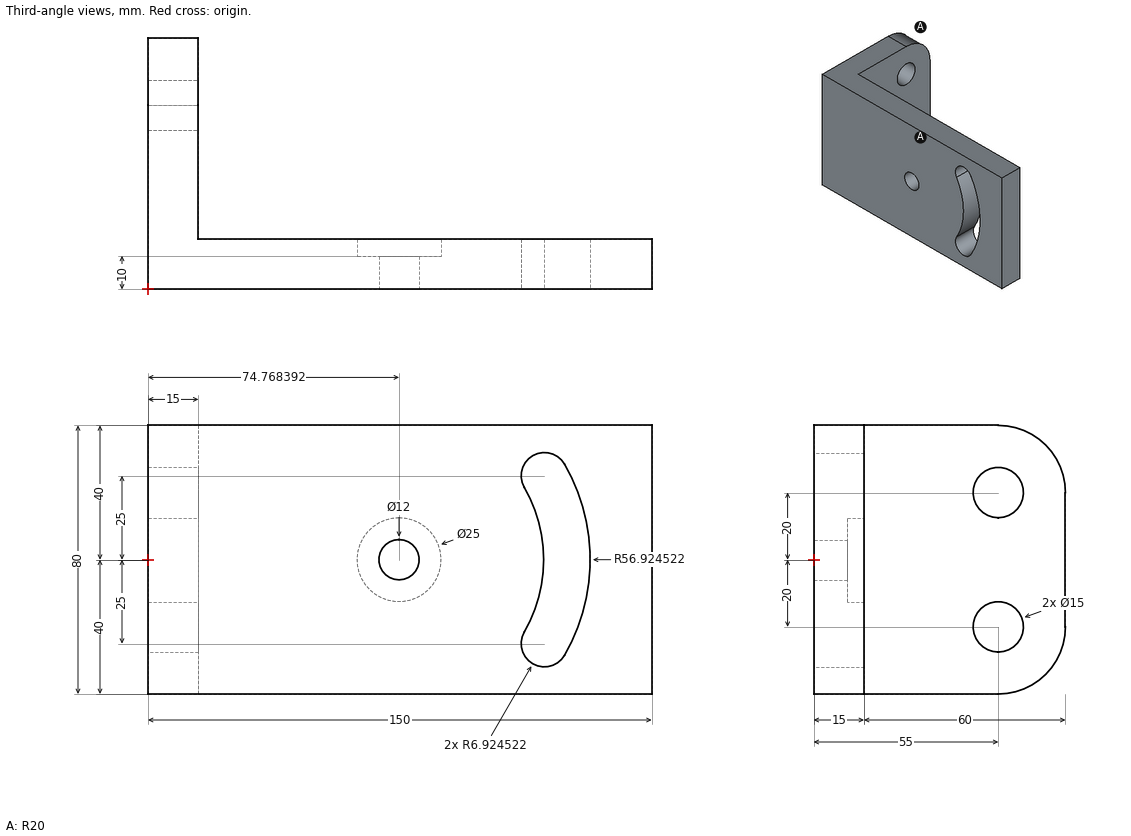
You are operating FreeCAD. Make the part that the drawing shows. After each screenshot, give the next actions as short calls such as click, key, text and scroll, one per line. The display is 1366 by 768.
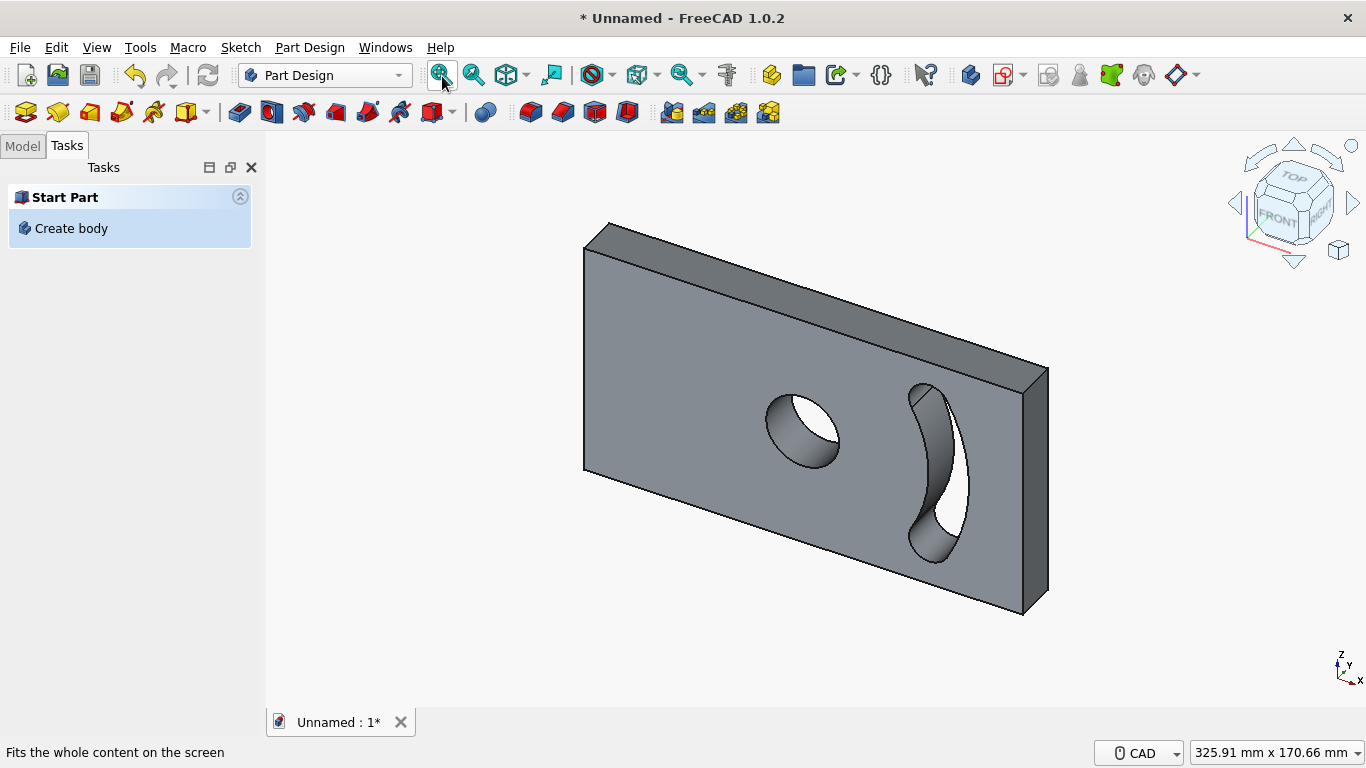
click(1004, 76)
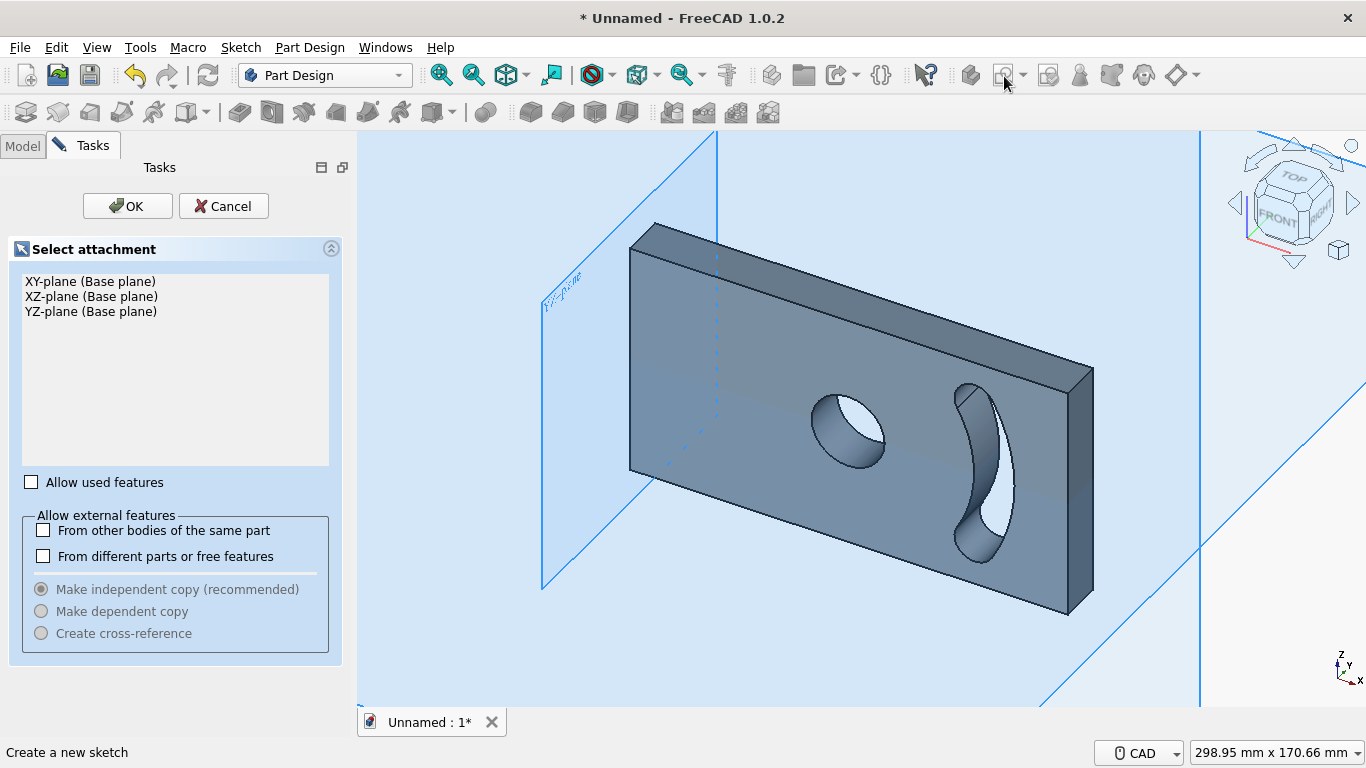
click(82, 296)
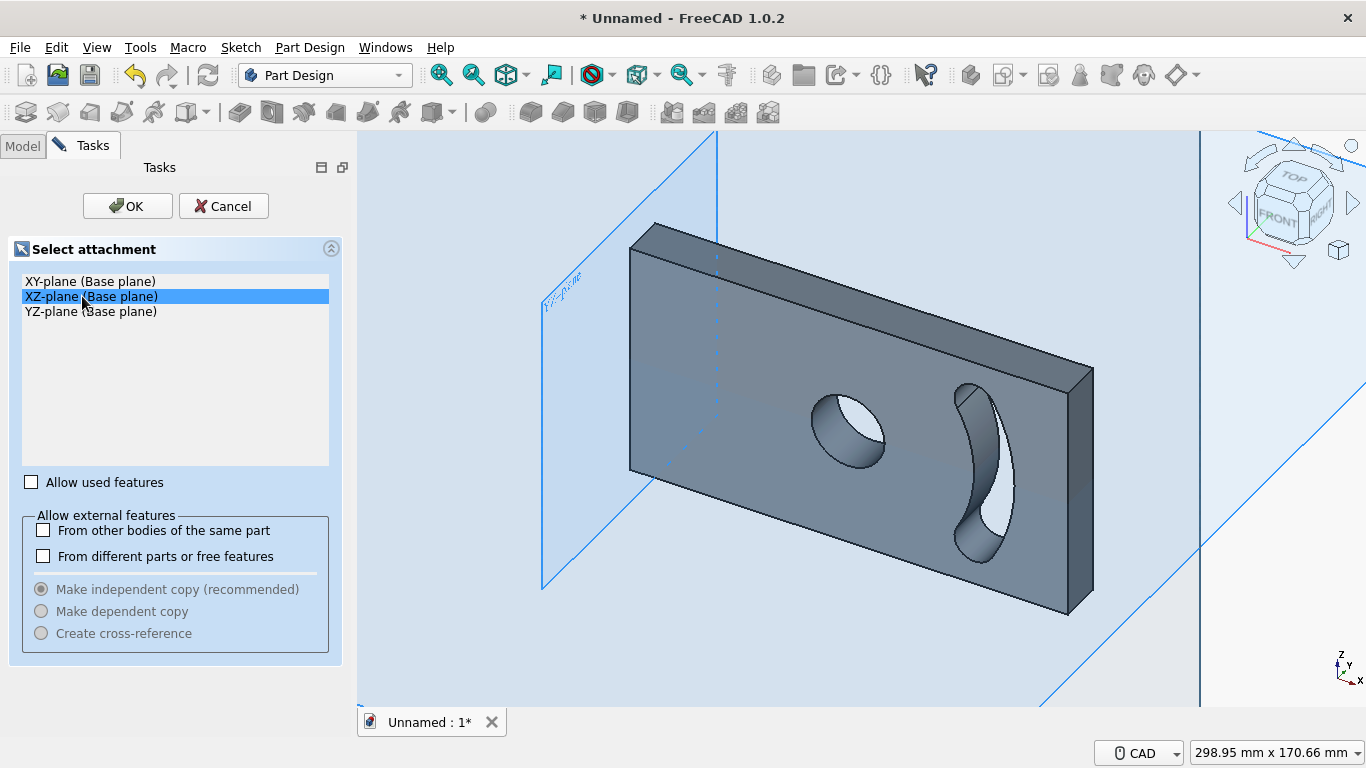
click(128, 206)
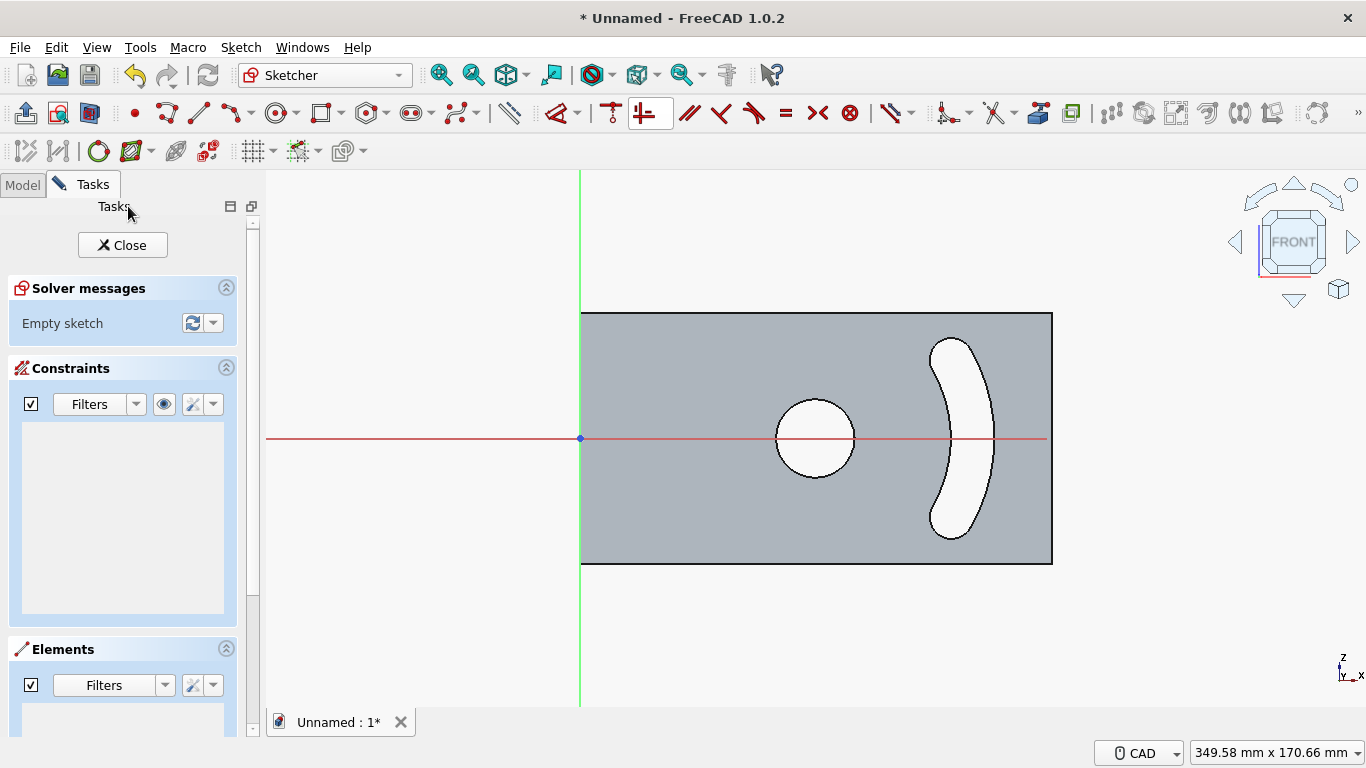
scroll(837, 439, up, 7)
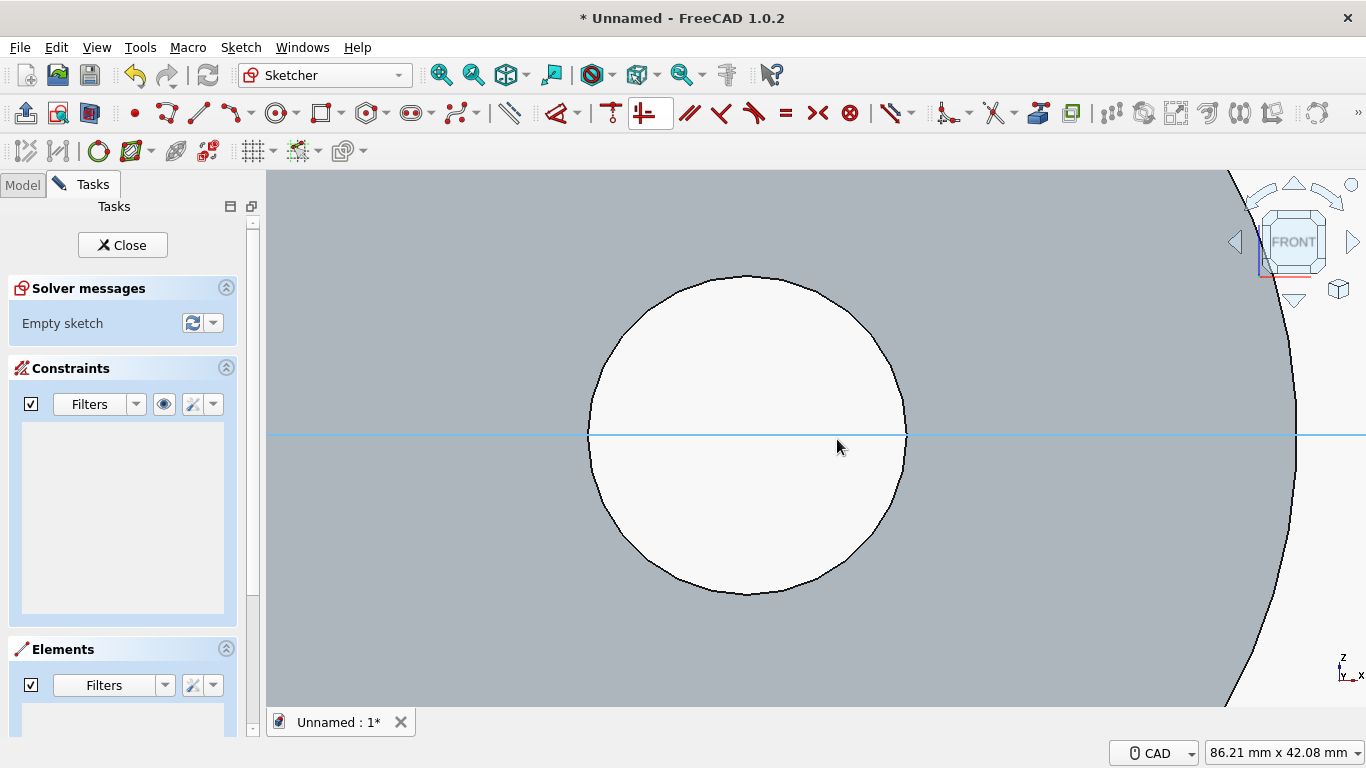
key(g)
key(c)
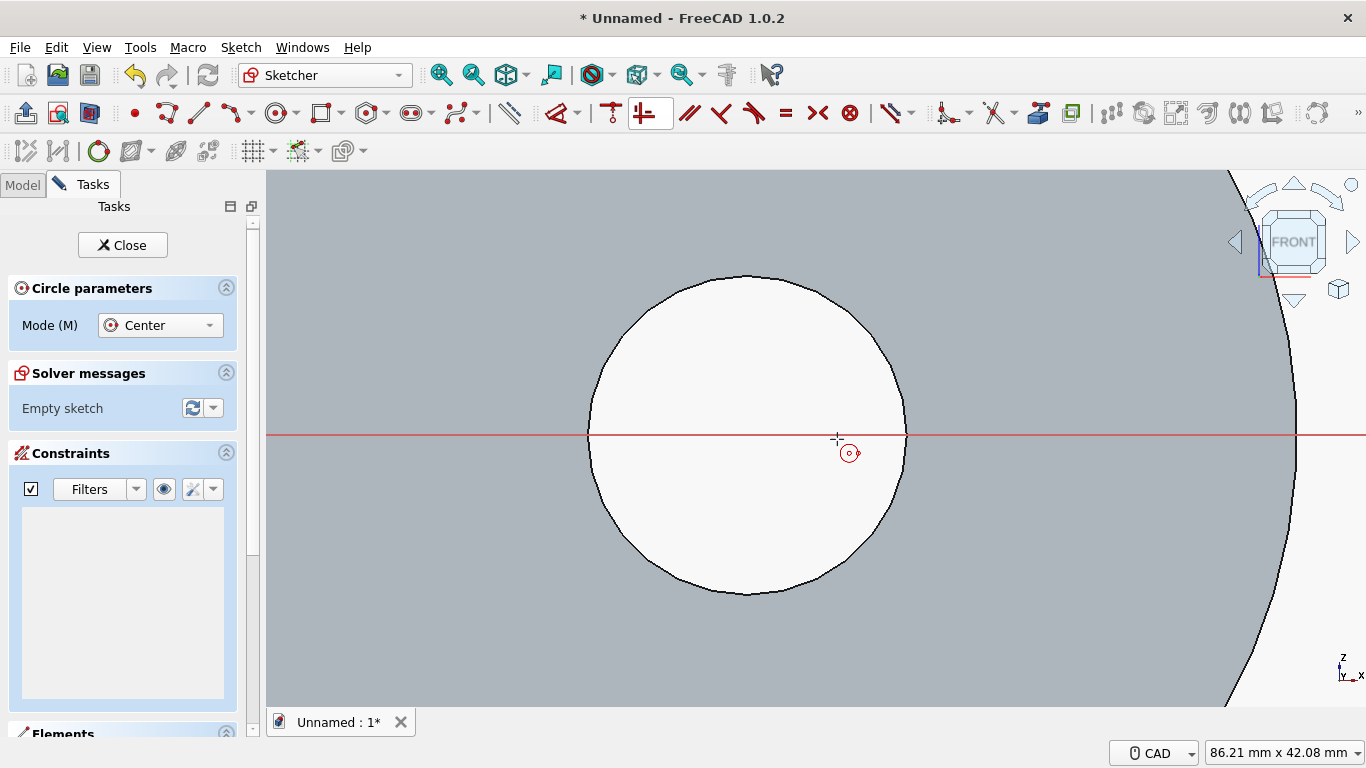
click(747, 435)
click(860, 323)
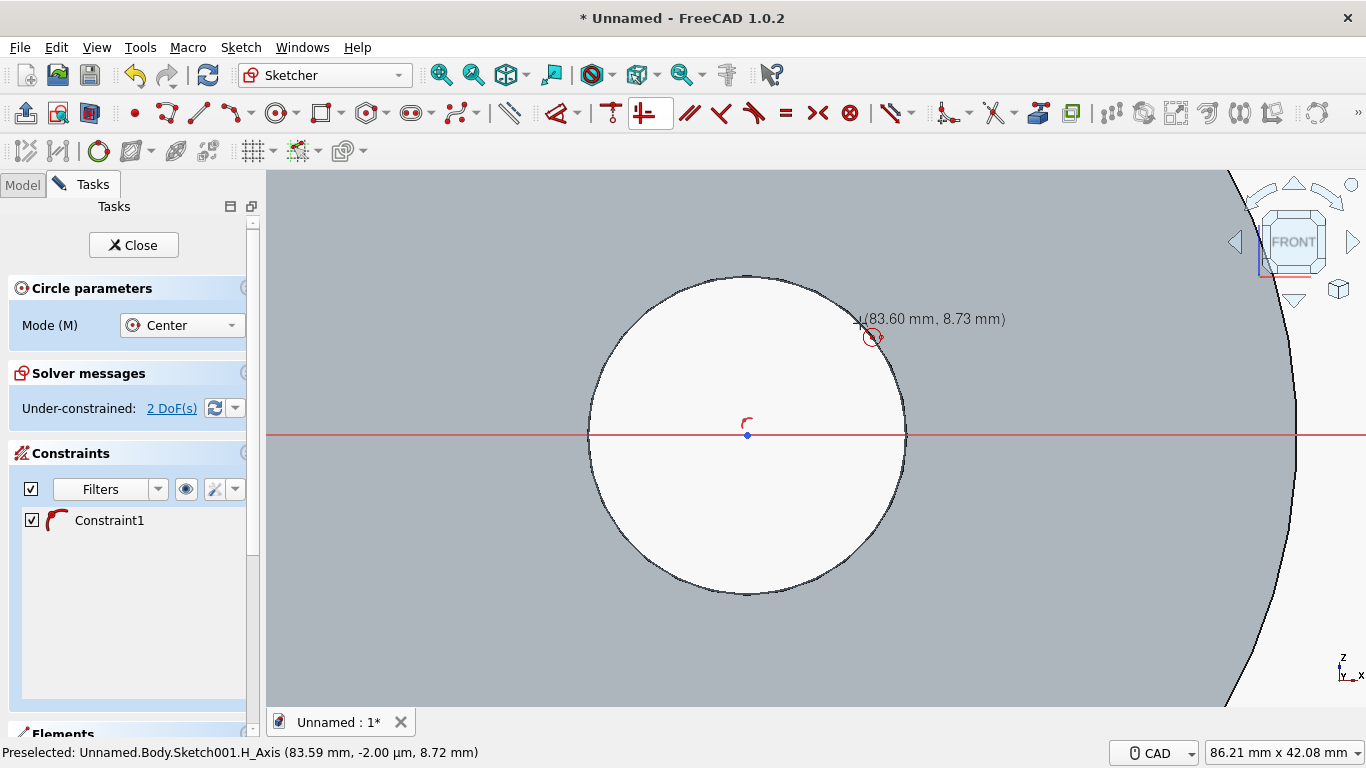
click(747, 435)
click(801, 381)
key(Escape)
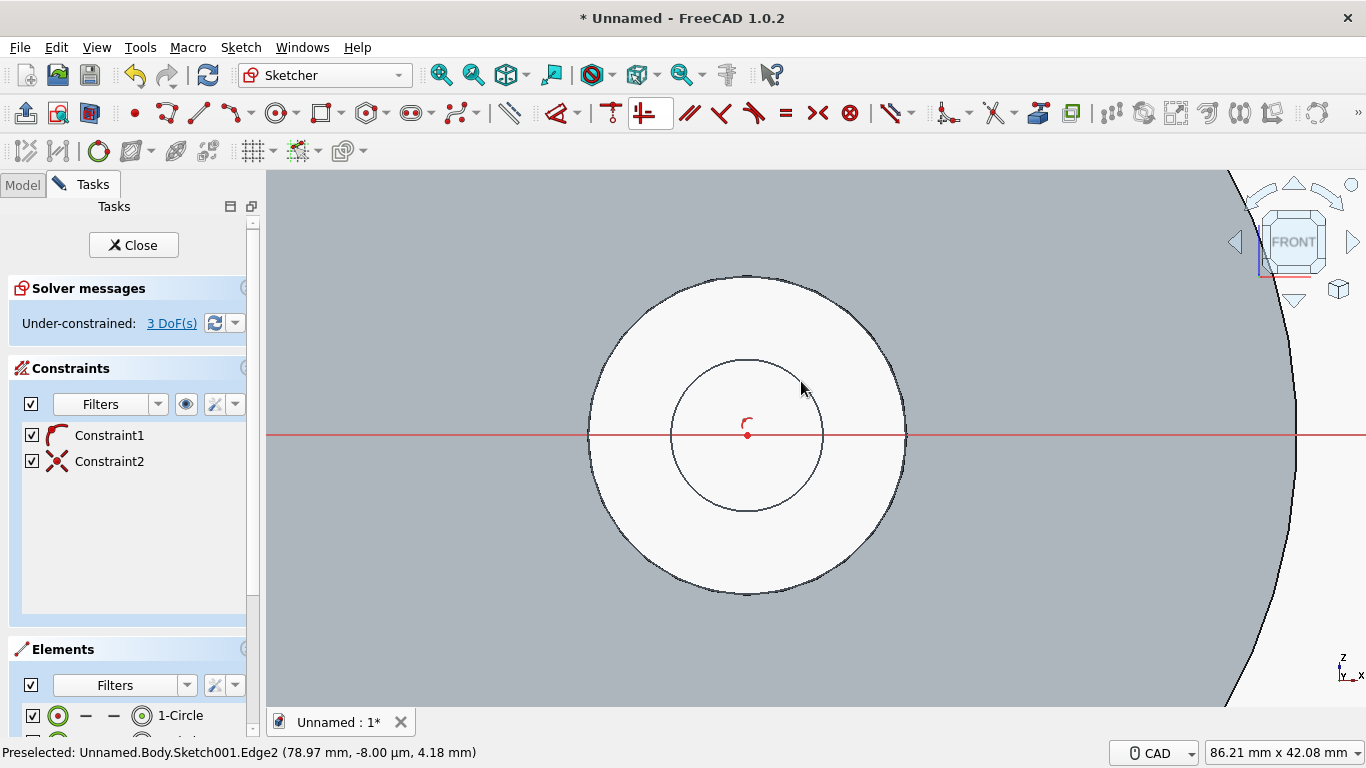
click(556, 114)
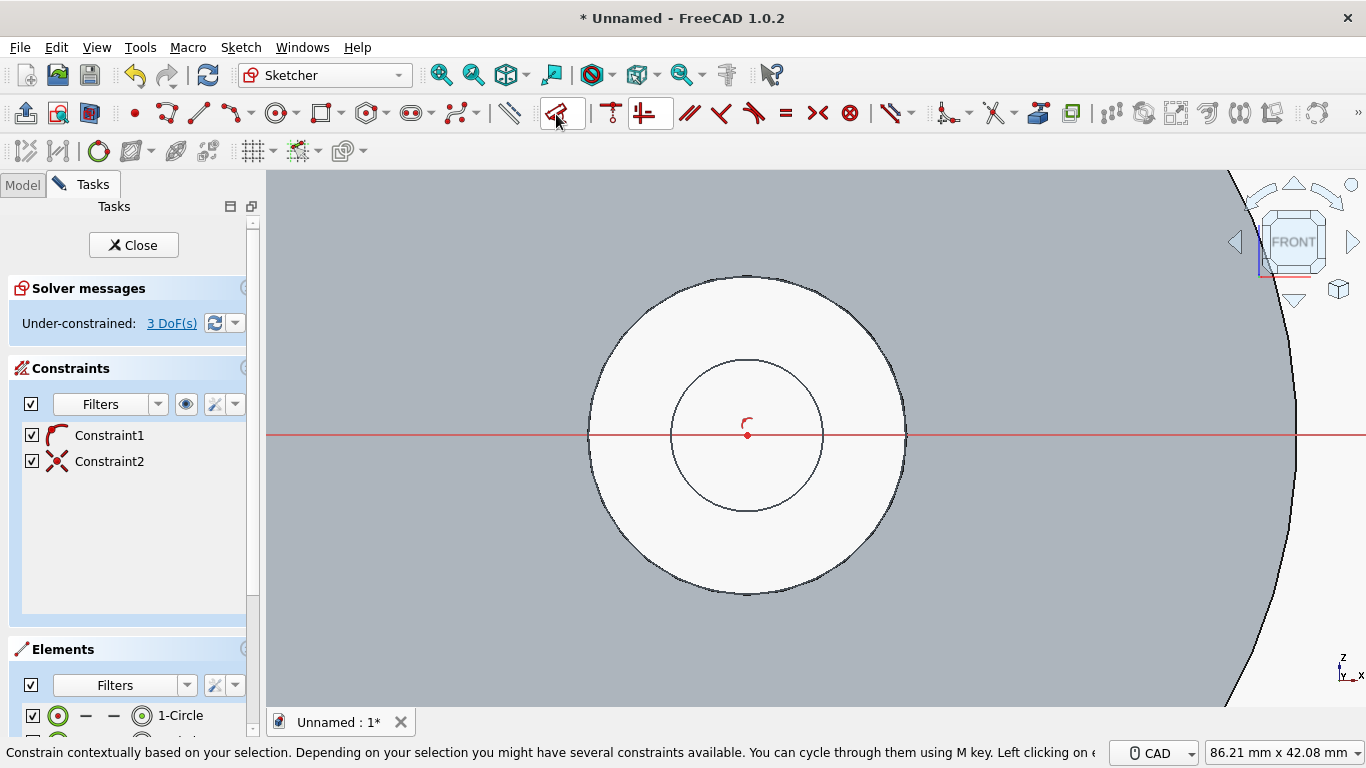
click(859, 323)
click(882, 300)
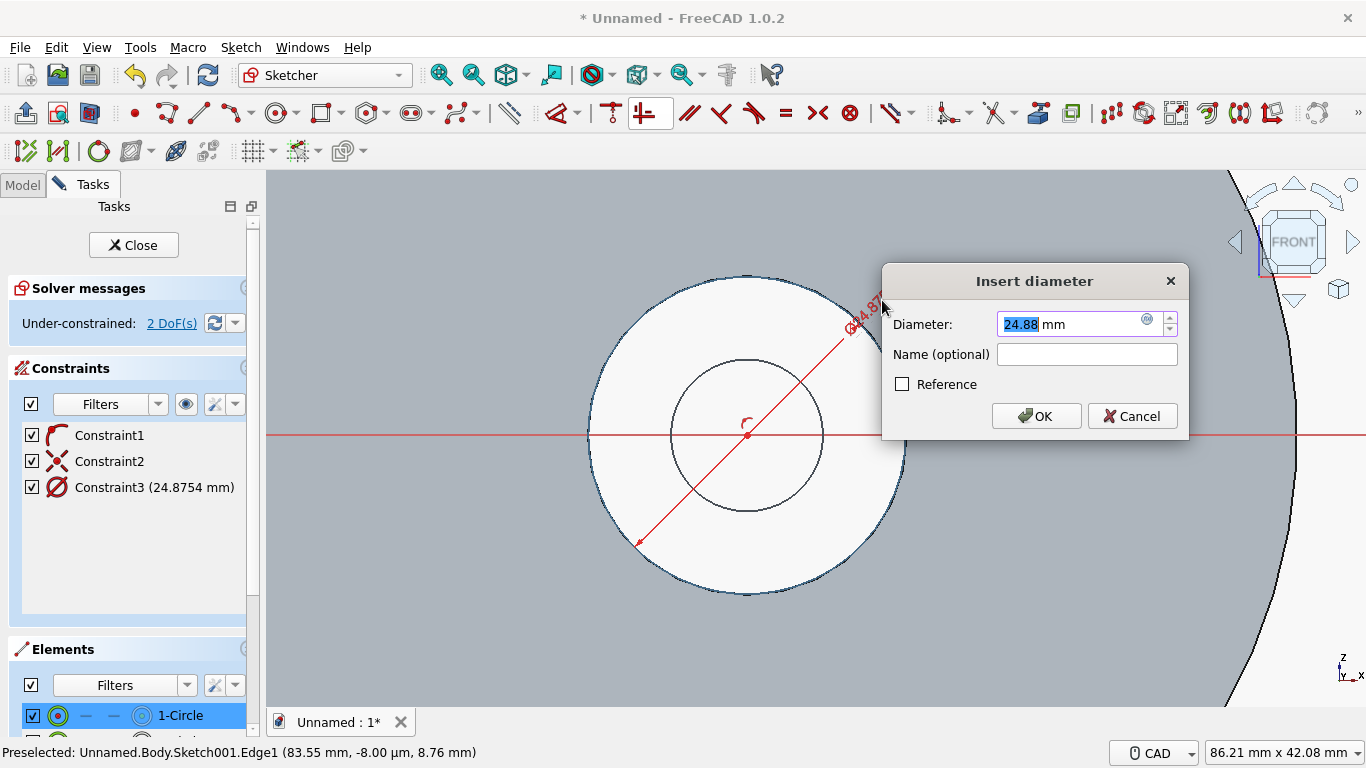
text(25)
key(Return)